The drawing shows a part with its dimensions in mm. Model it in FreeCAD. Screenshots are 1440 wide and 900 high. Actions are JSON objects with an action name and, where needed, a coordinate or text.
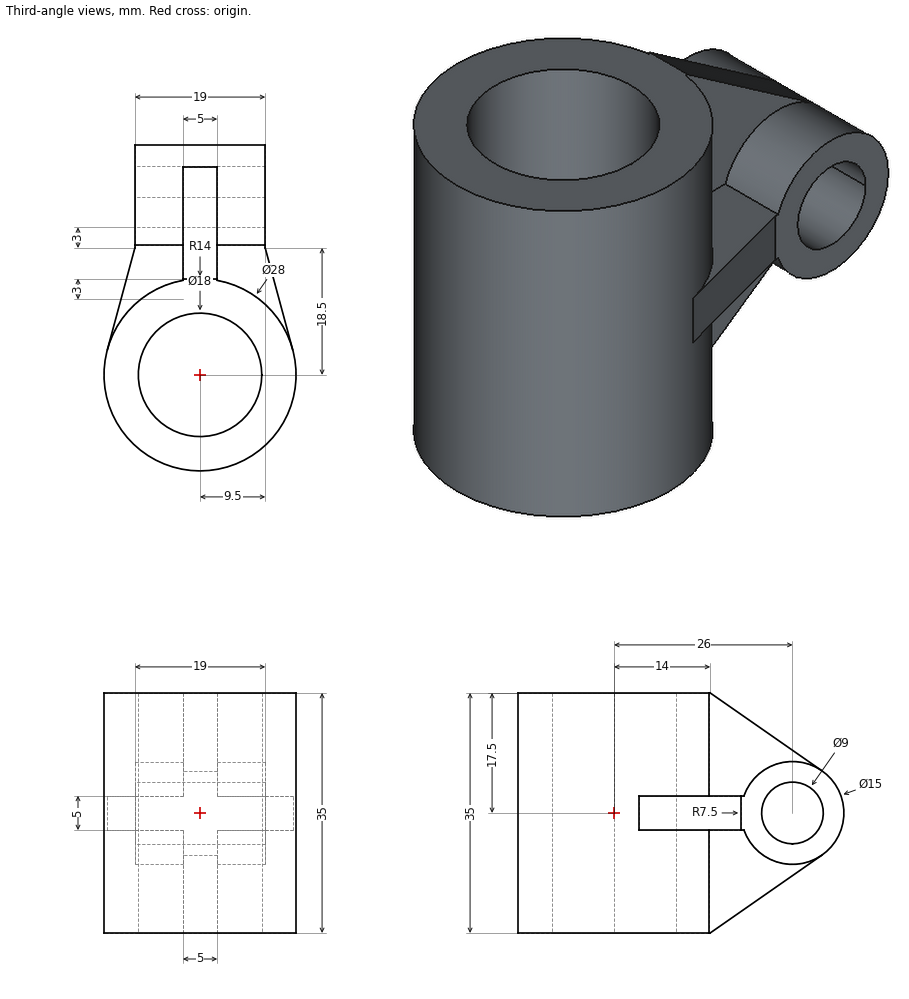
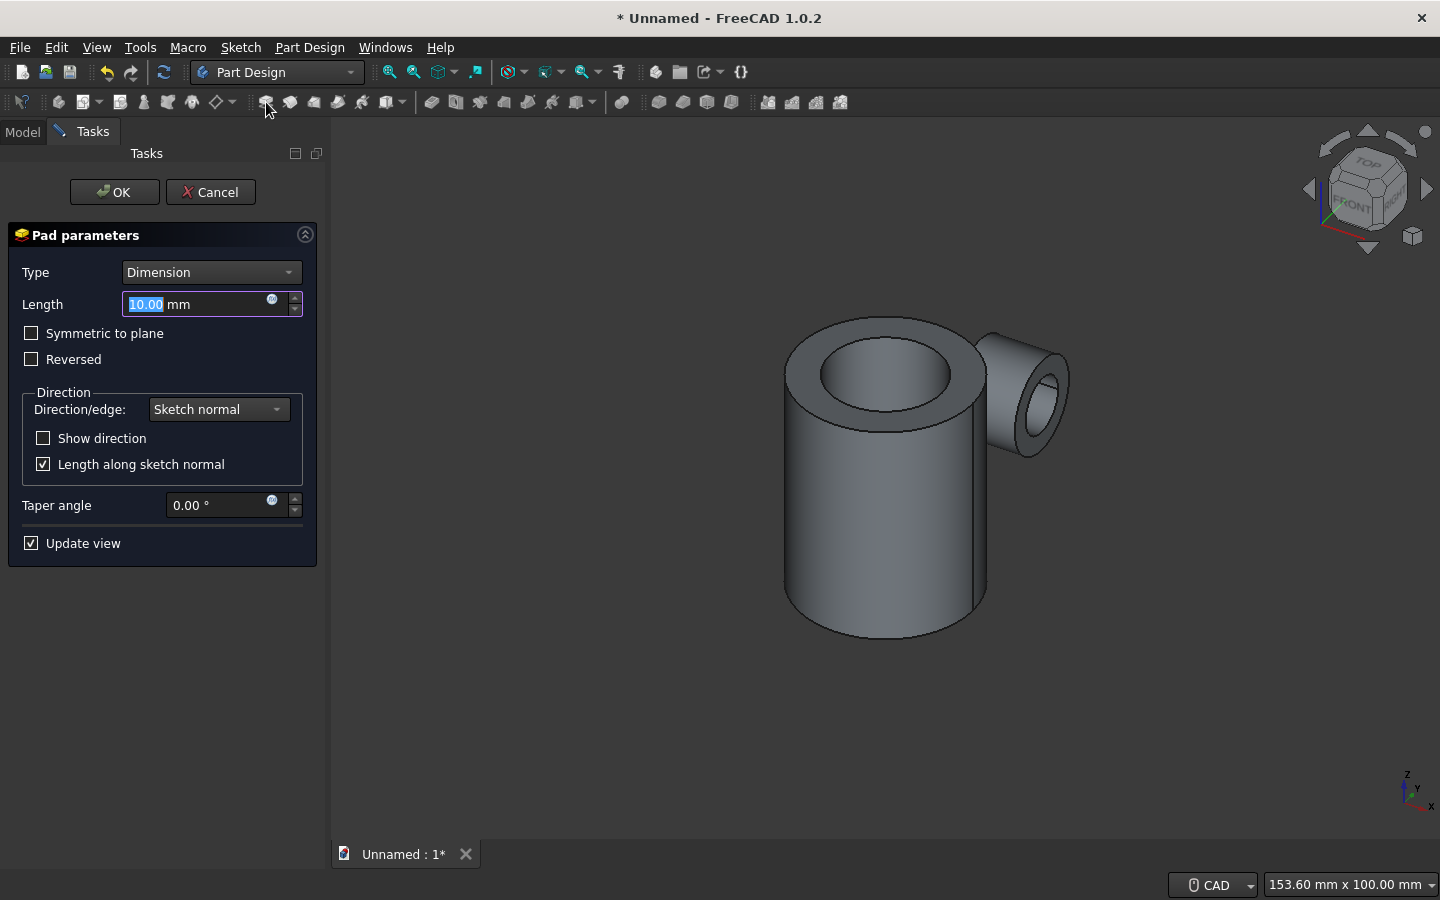
{"action": "type", "text": "19"}
{"action": "key", "text": "Tab"}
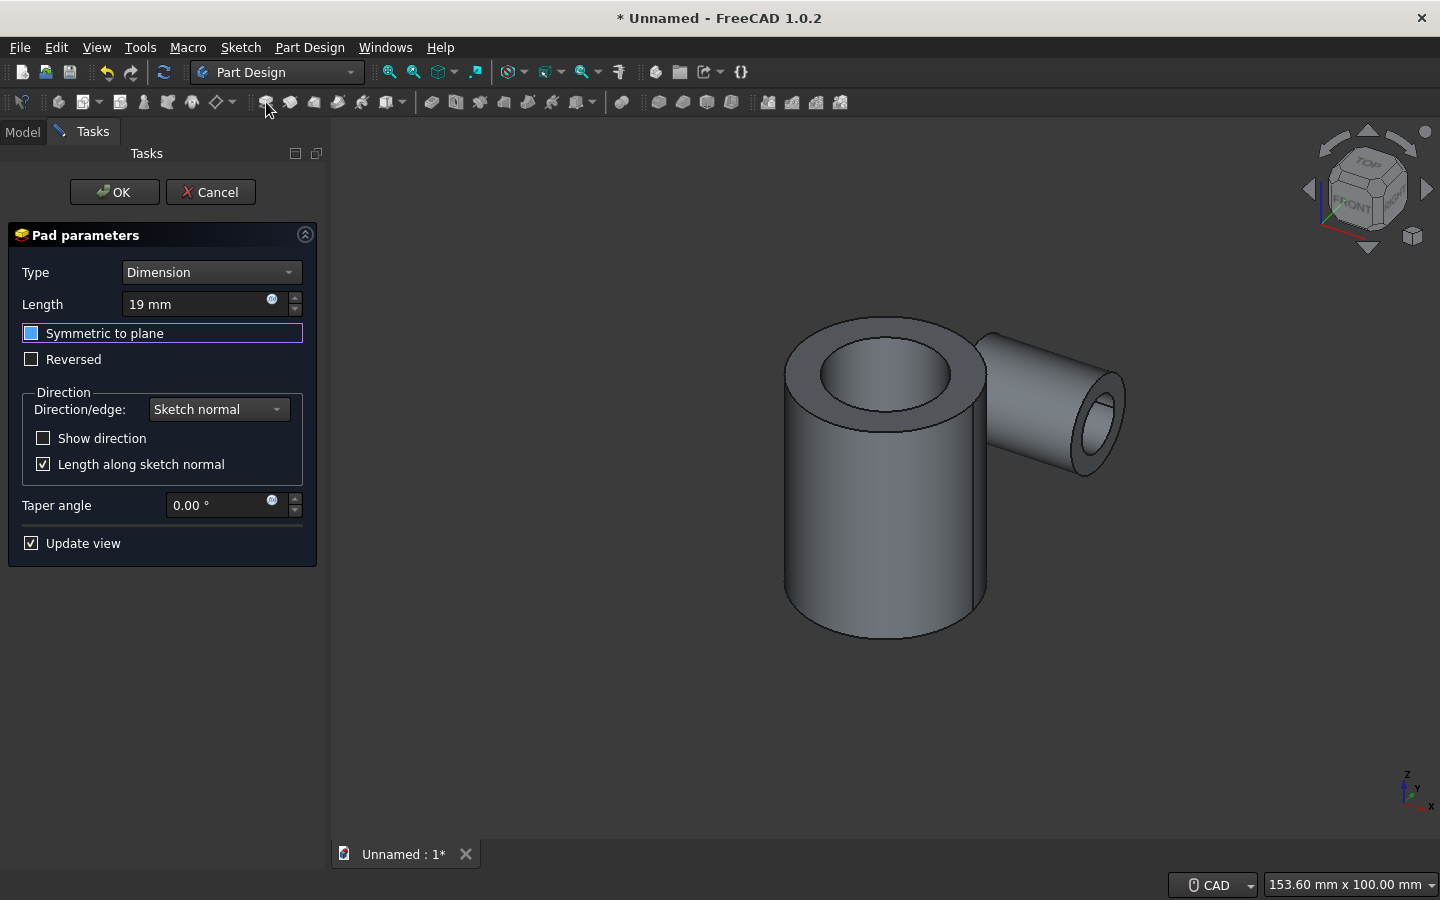
{"action": "left_click", "coordinate": [30, 333]}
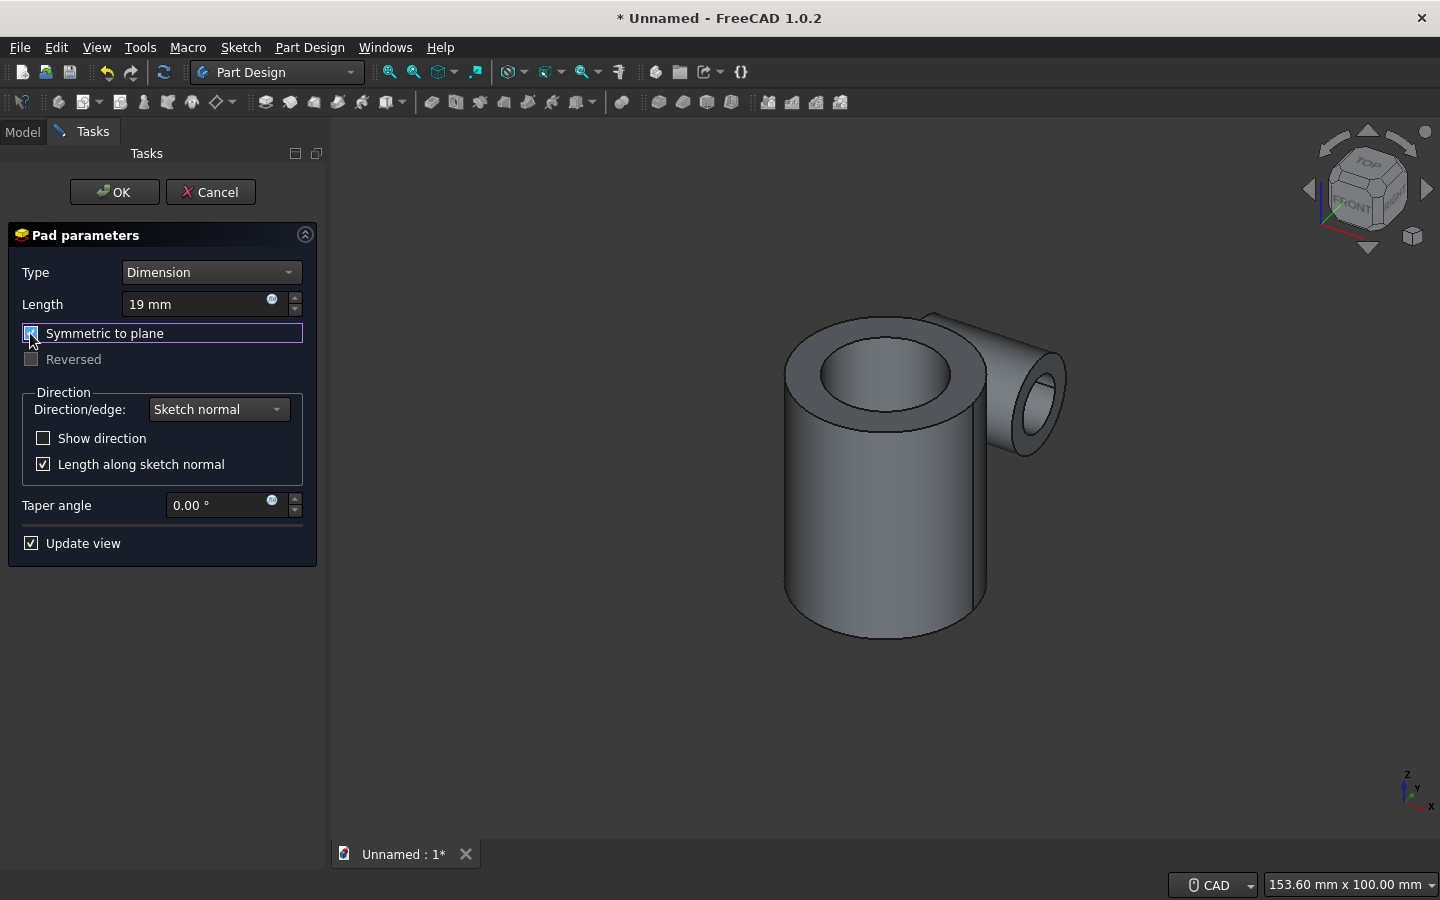
{"action": "left_click", "coordinate": [115, 192]}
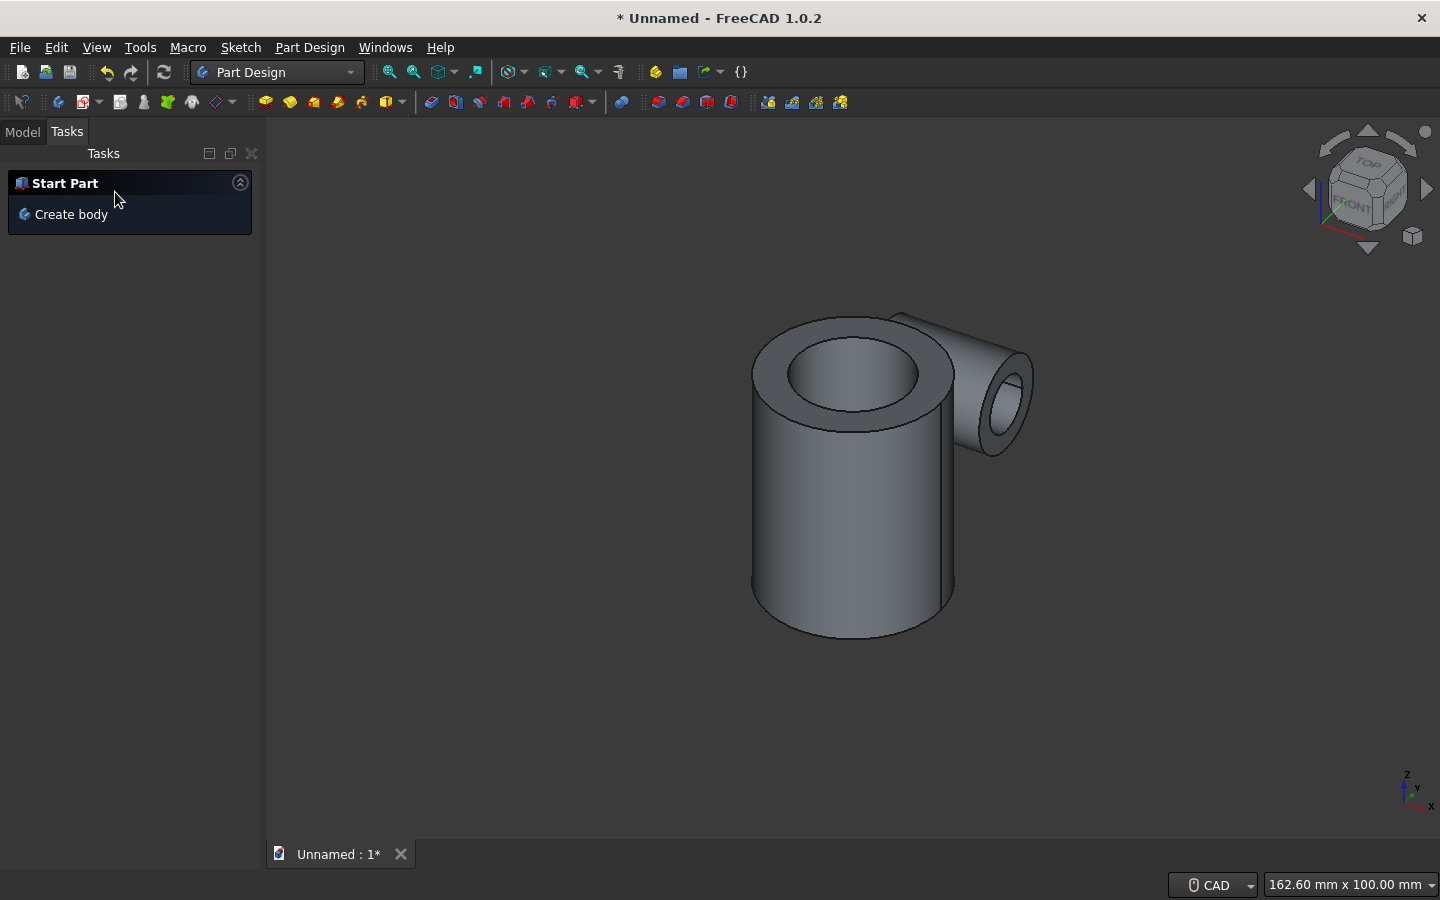
{"action": "key", "text": "v f"}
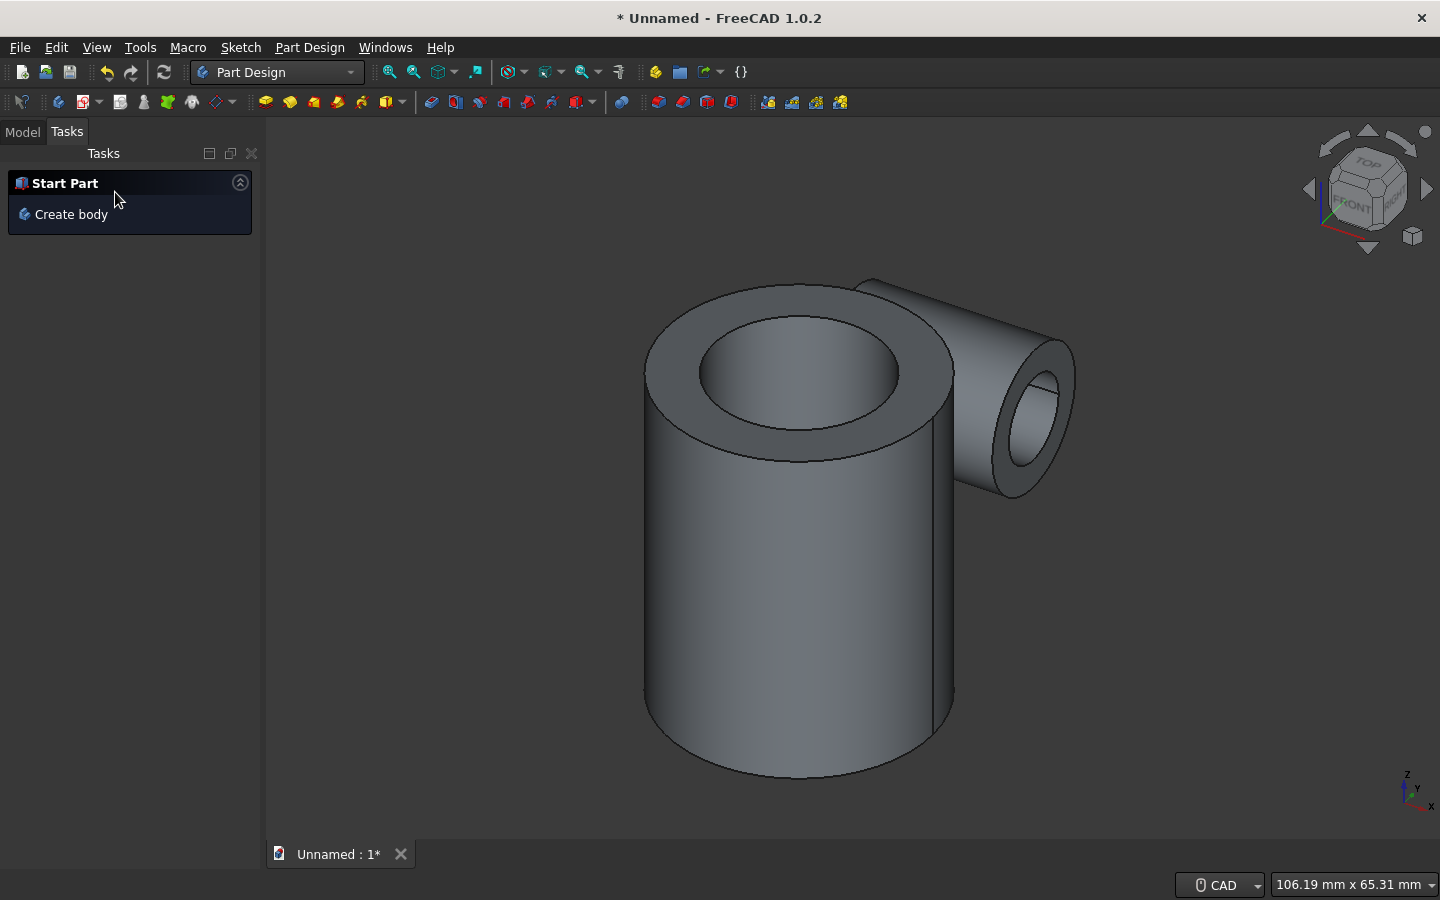
{"action": "left_click", "coordinate": [84, 102]}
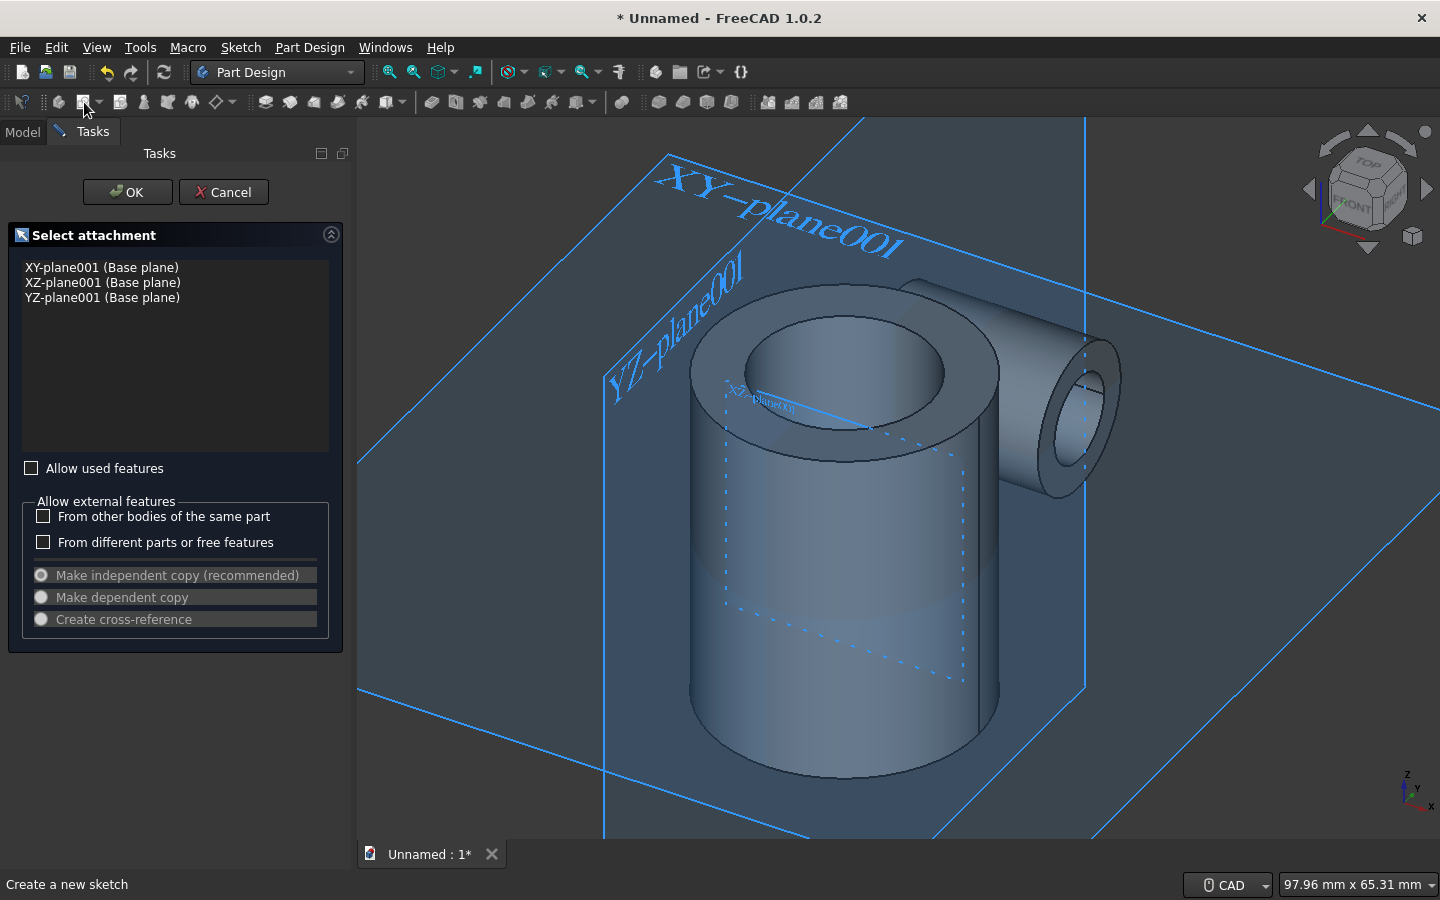
{"action": "left_click", "coordinate": [82, 298]}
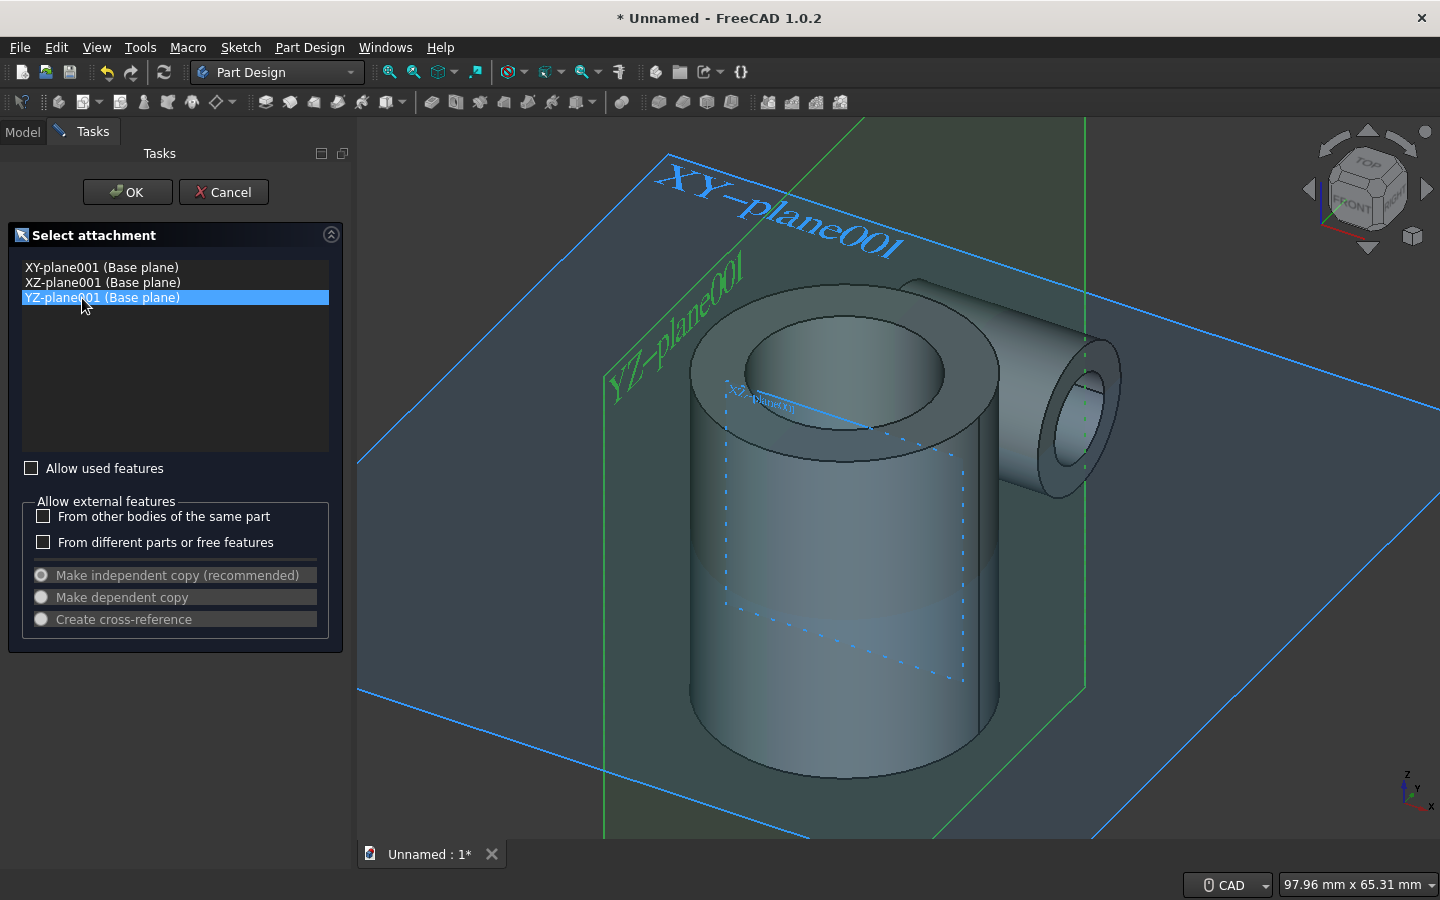
{"action": "left_click", "coordinate": [128, 192]}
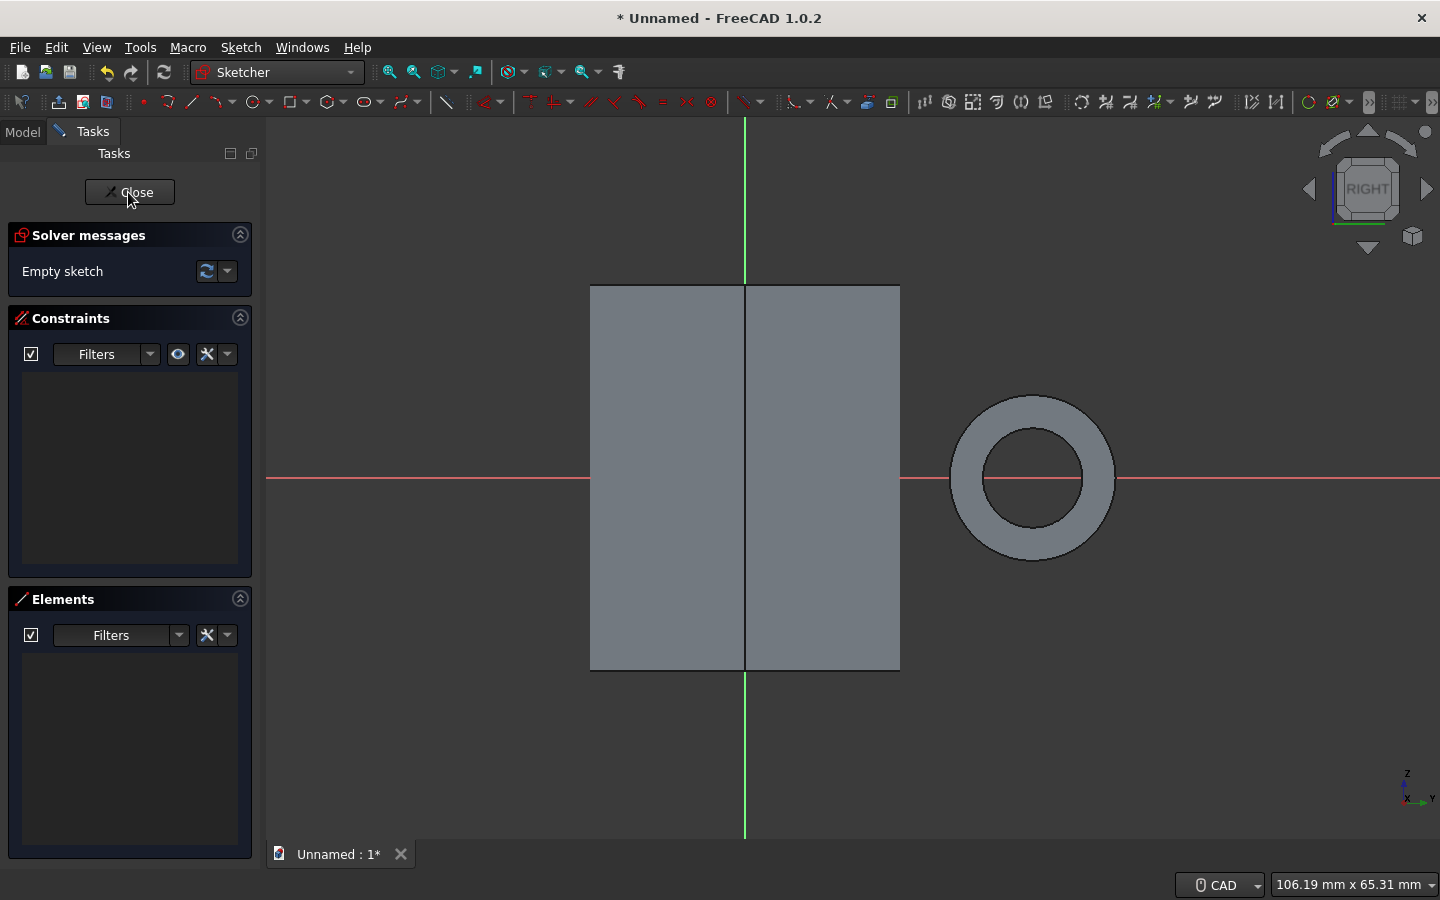
{"action": "key", "text": "q s"}